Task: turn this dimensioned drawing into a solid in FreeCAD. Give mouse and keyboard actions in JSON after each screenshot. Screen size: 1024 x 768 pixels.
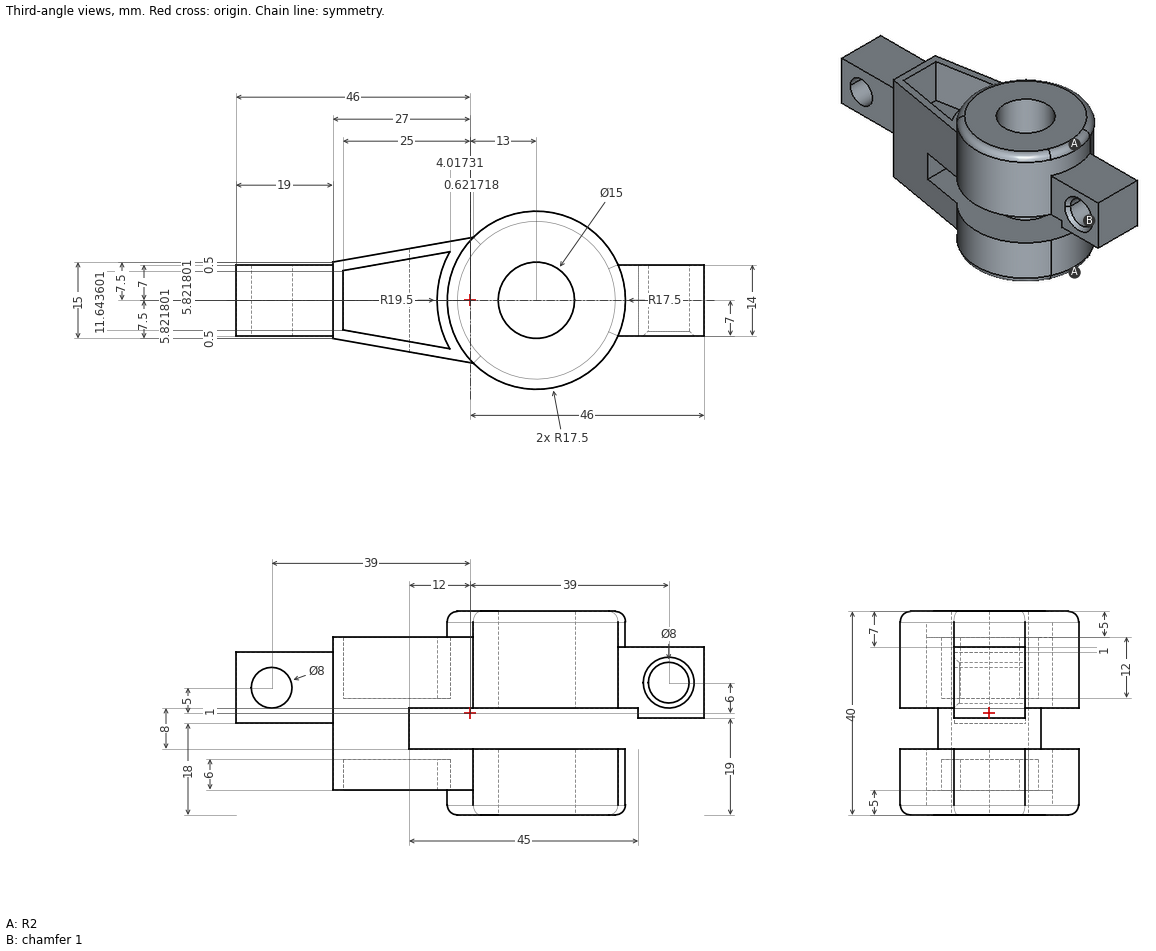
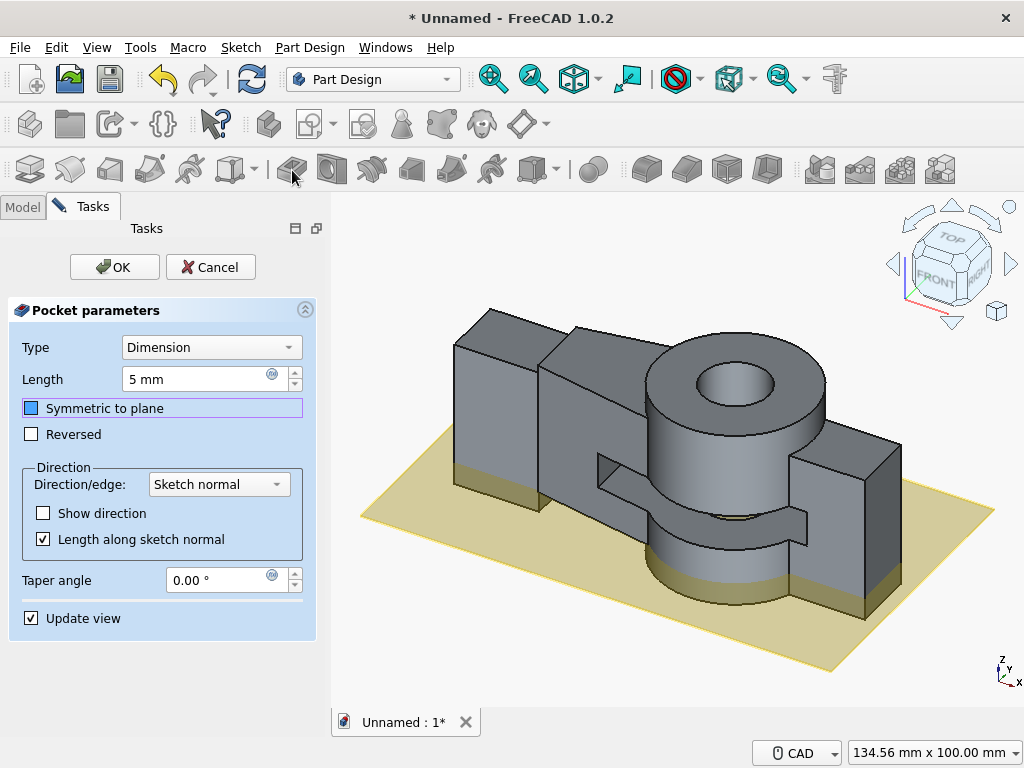
{"action": "left_click", "coordinate": [115, 267]}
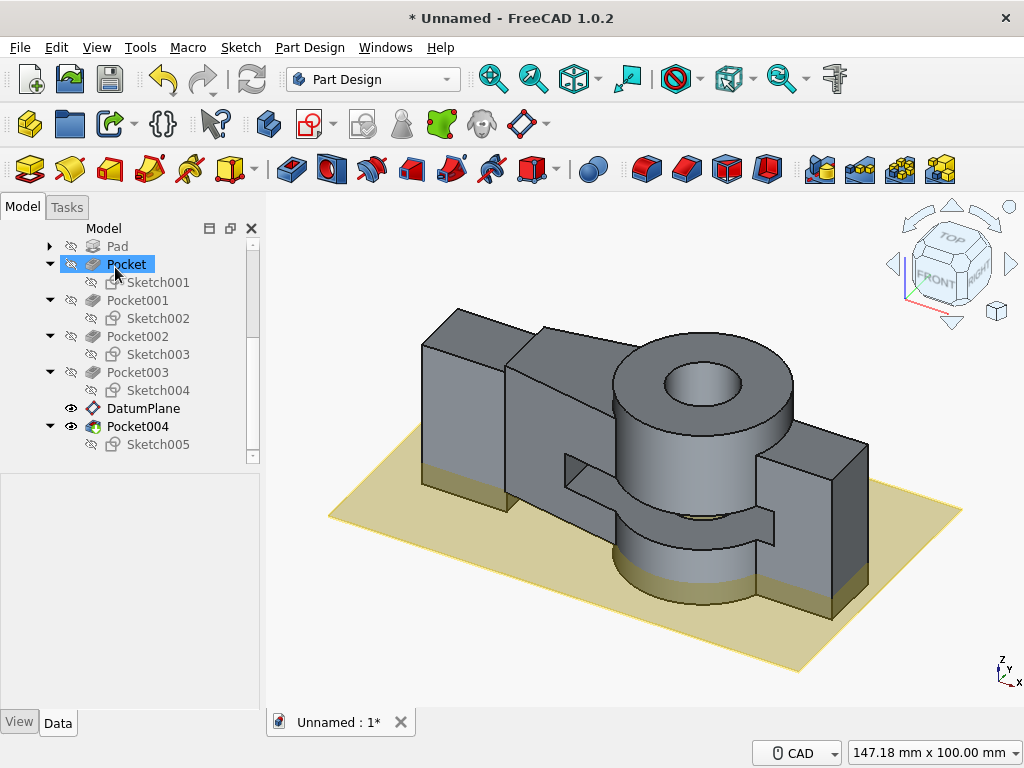
{"action": "left_click", "coordinate": [116, 408]}
{"action": "key", "text": "space"}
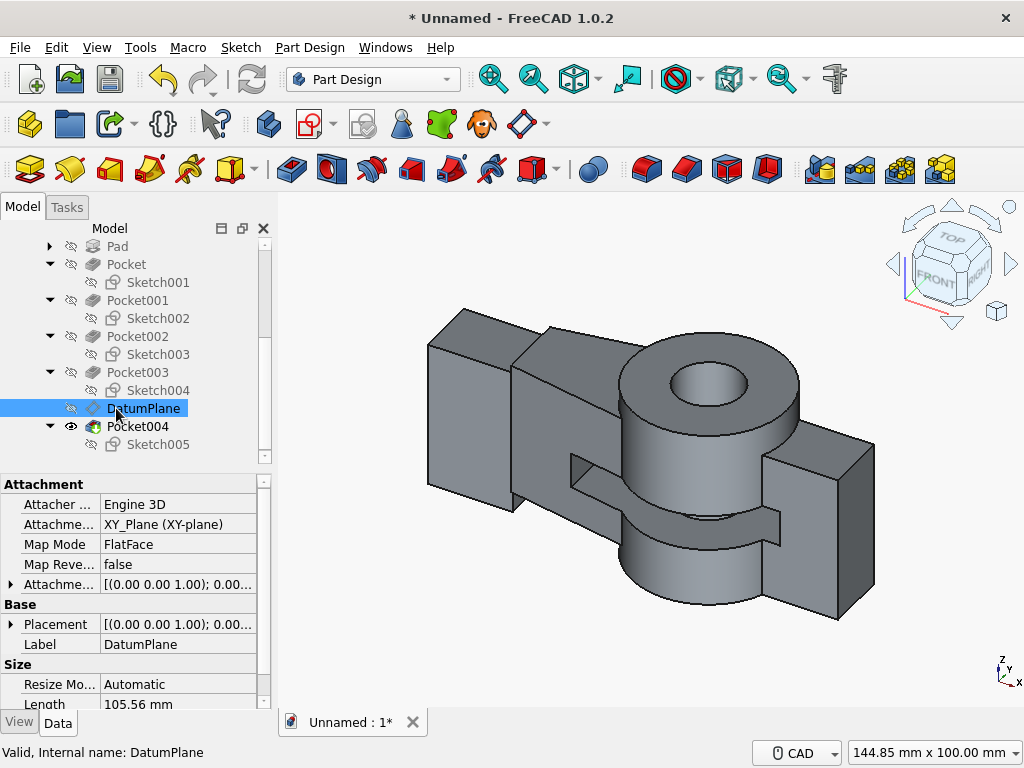
{"action": "key", "text": "5"}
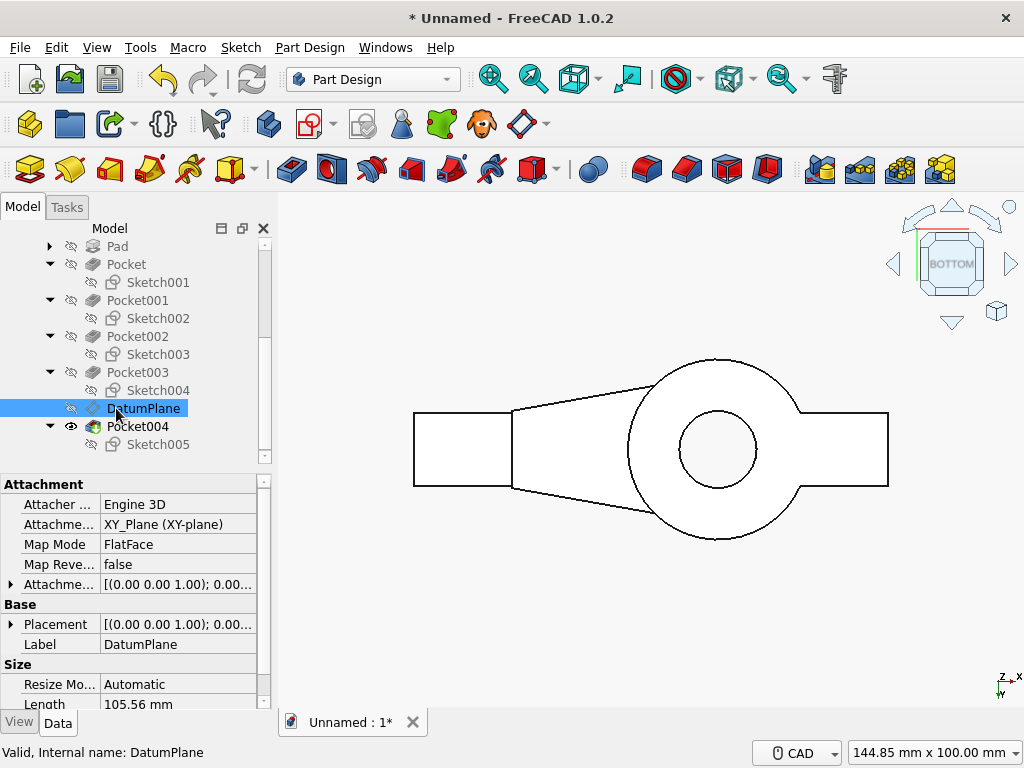
{"action": "left_click", "coordinate": [795, 448]}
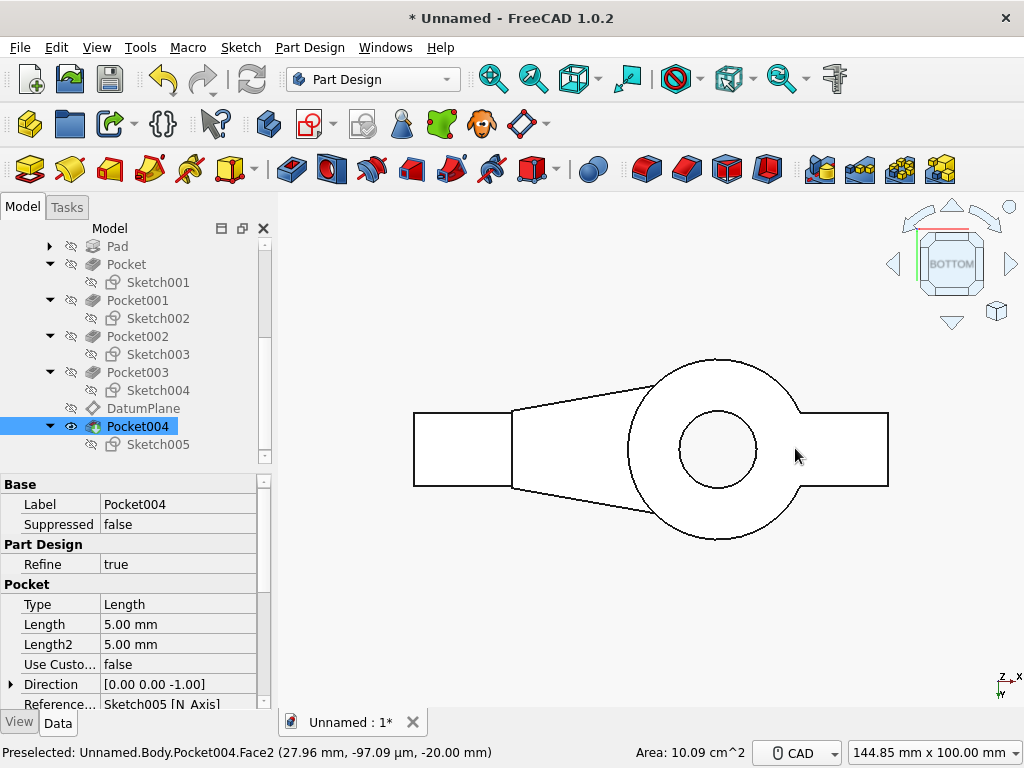
{"action": "left_click", "coordinate": [310, 124]}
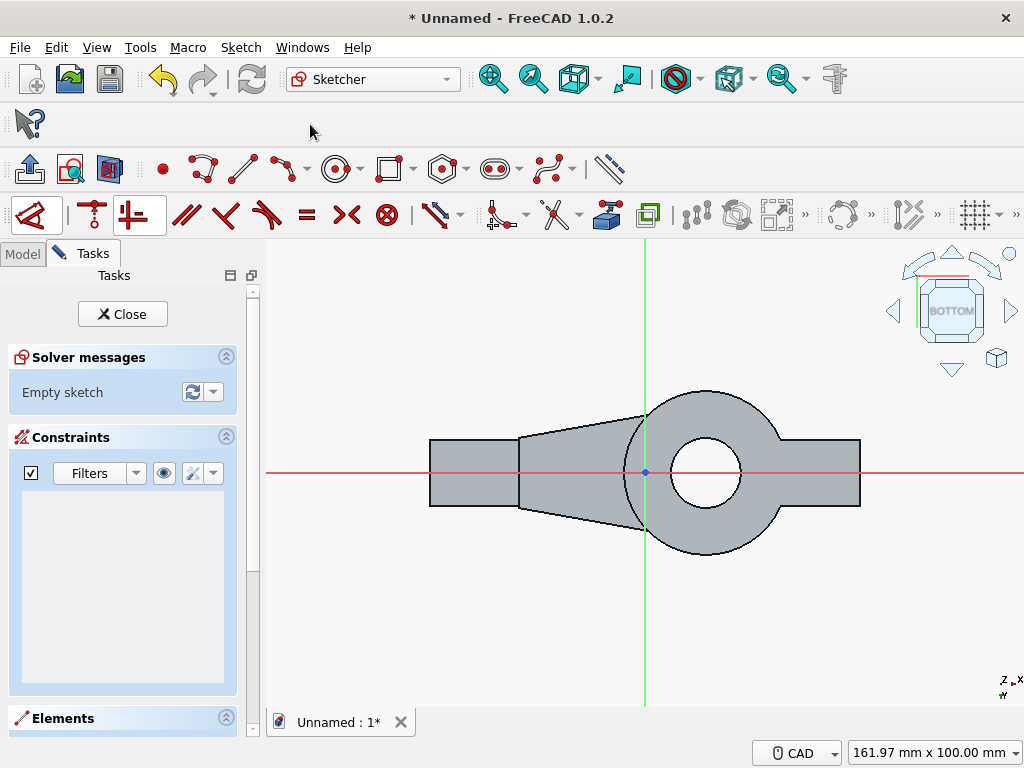
{"action": "scroll", "coordinate": [490, 473], "scroll_direction": "up", "scroll_amount": 3}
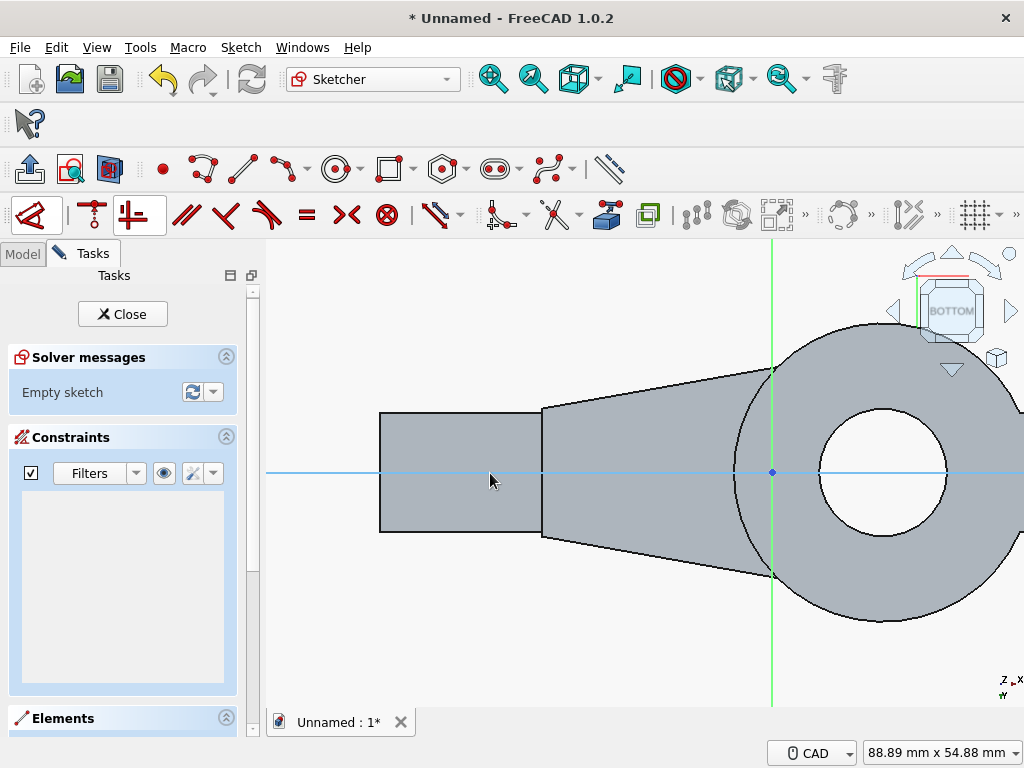
{"action": "left_click", "coordinate": [390, 170]}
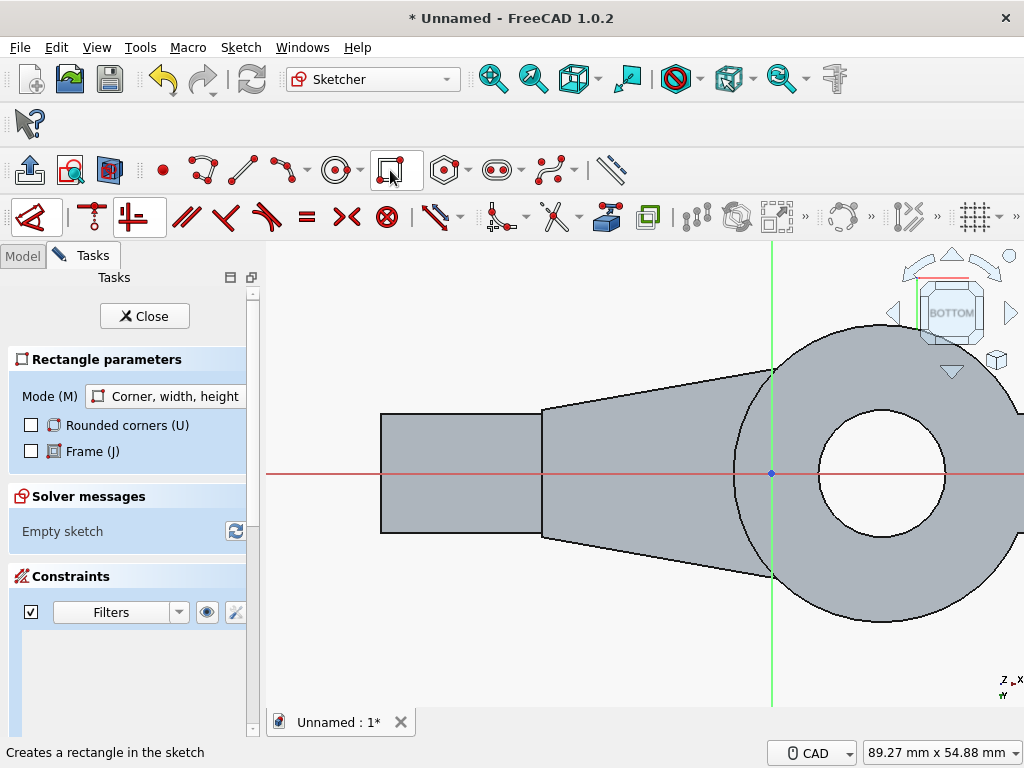
{"action": "left_click", "coordinate": [381, 414]}
{"action": "left_click", "coordinate": [542, 533]}
{"action": "key", "text": "Escape"}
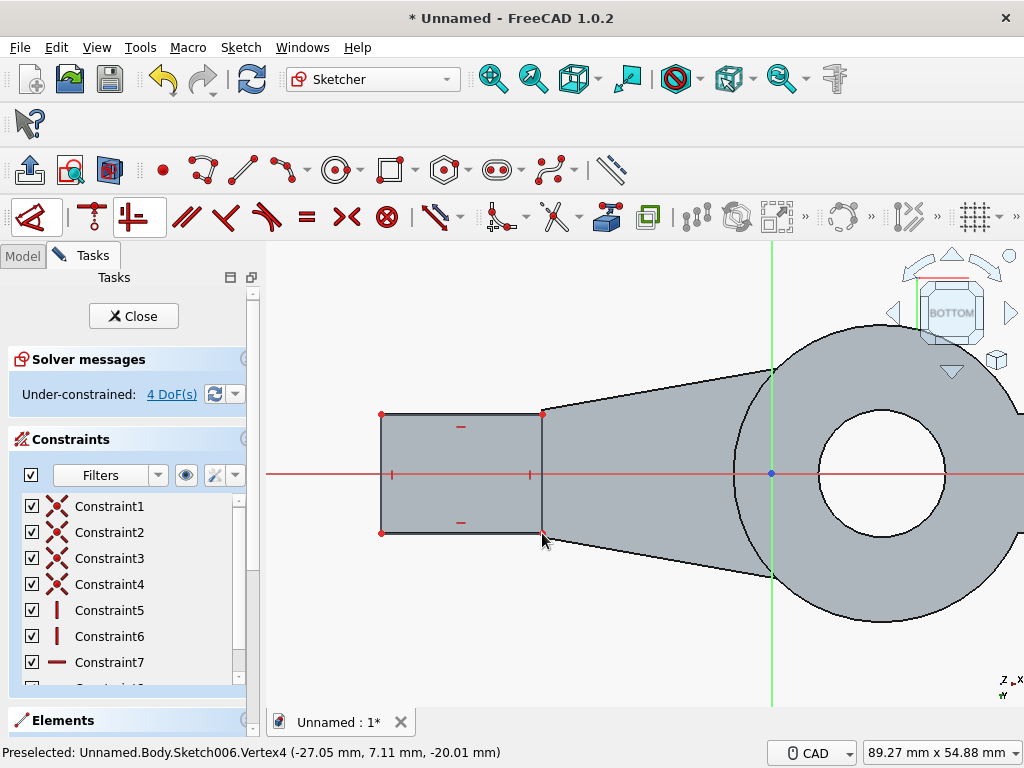
{"action": "left_click", "coordinate": [381, 451]}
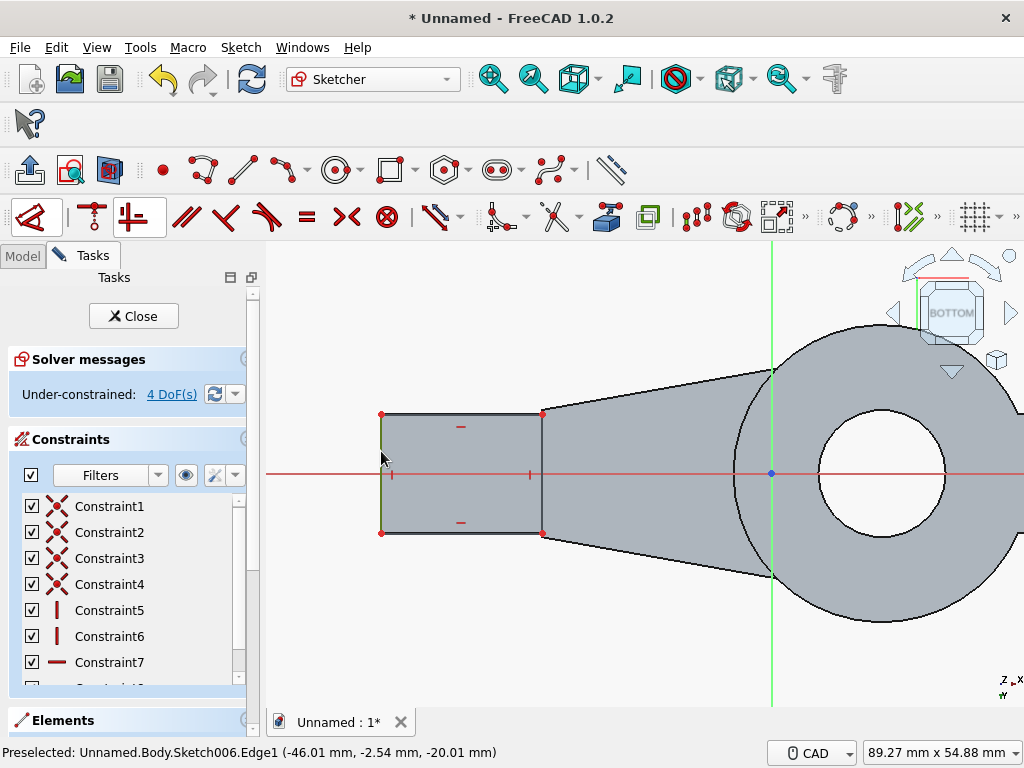
{"action": "left_click", "coordinate": [56, 218]}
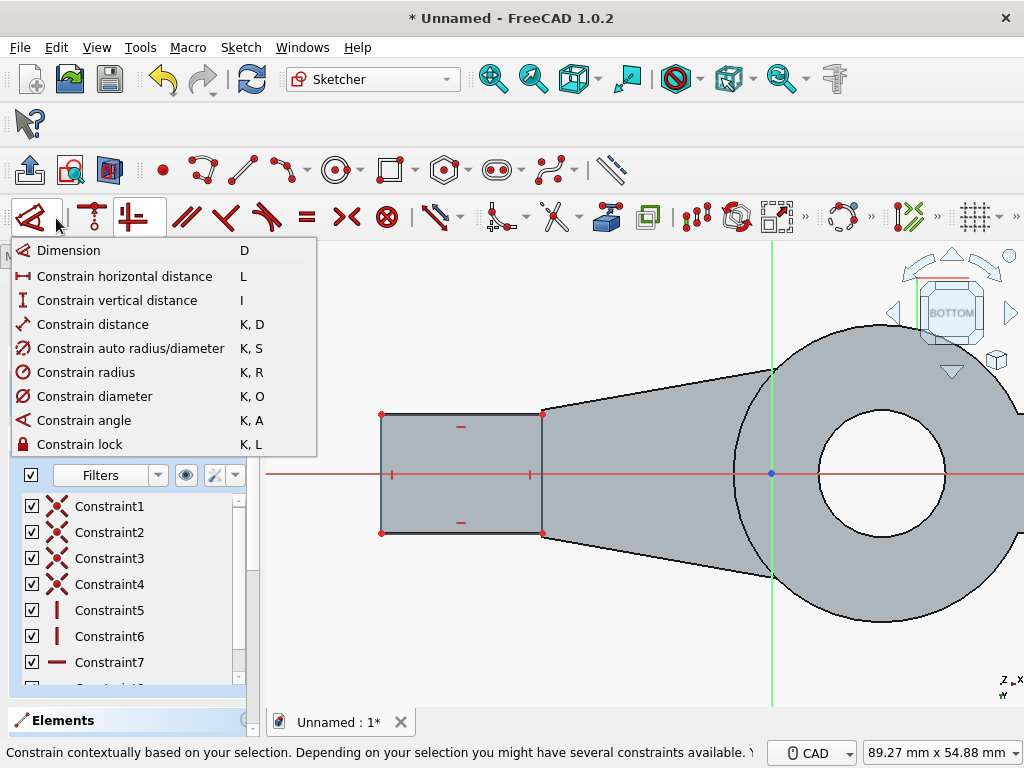
{"action": "left_click", "coordinate": [164, 300]}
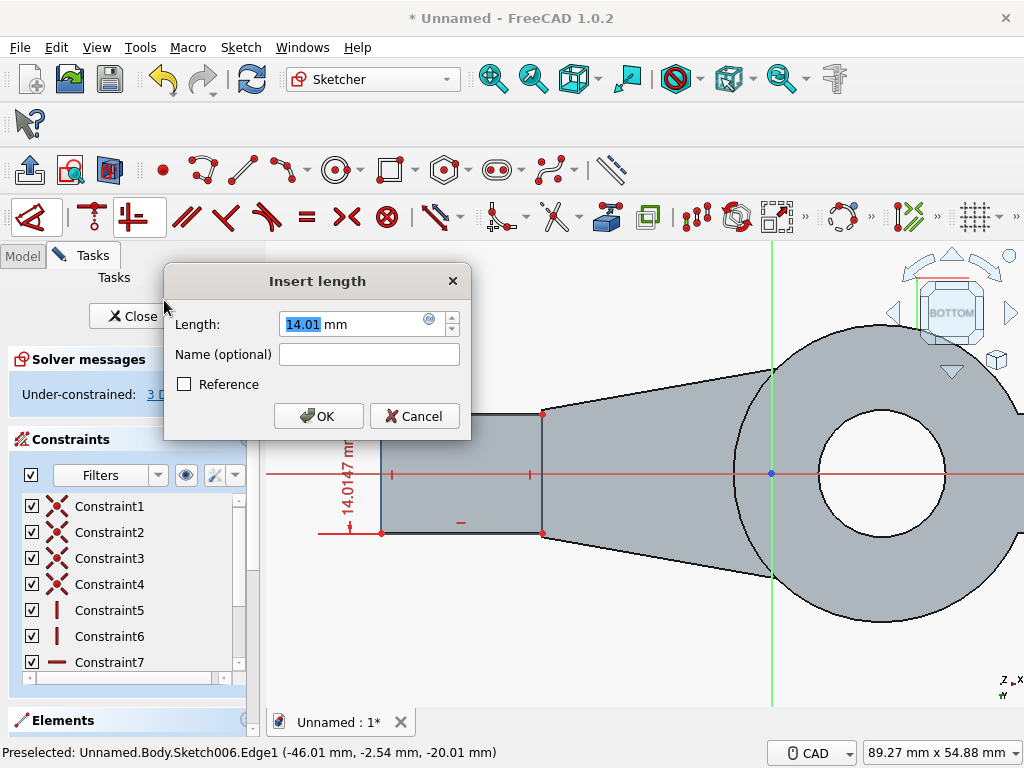
{"action": "type", "text": "14"}
{"action": "key", "text": "Return"}